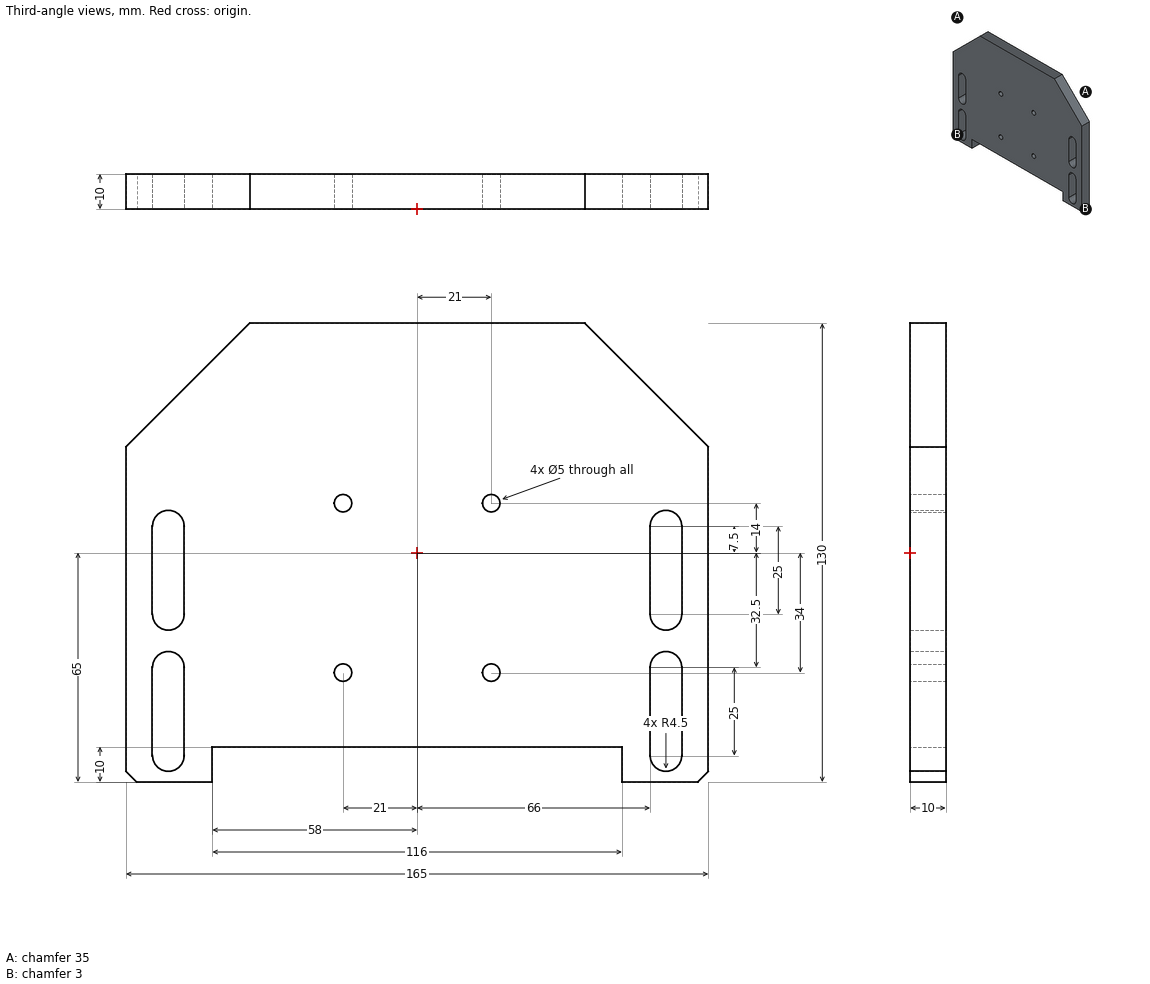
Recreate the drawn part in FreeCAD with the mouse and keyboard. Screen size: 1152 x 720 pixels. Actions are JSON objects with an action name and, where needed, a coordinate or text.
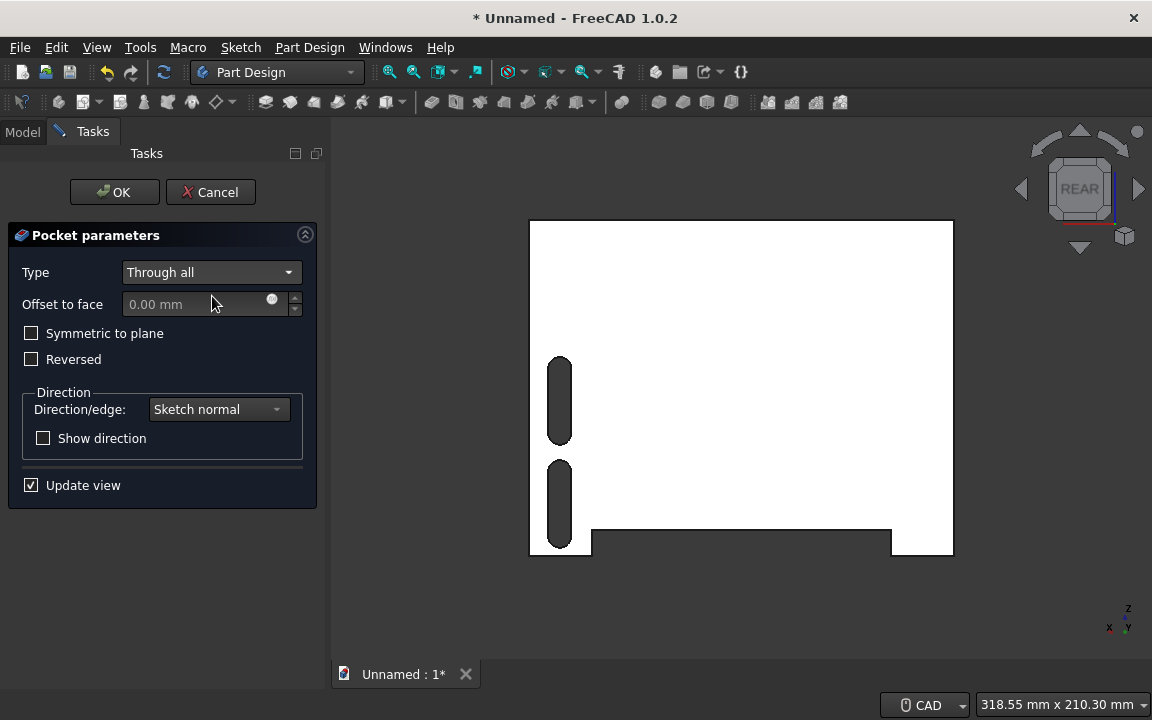
{"action": "left_click", "coordinate": [115, 192]}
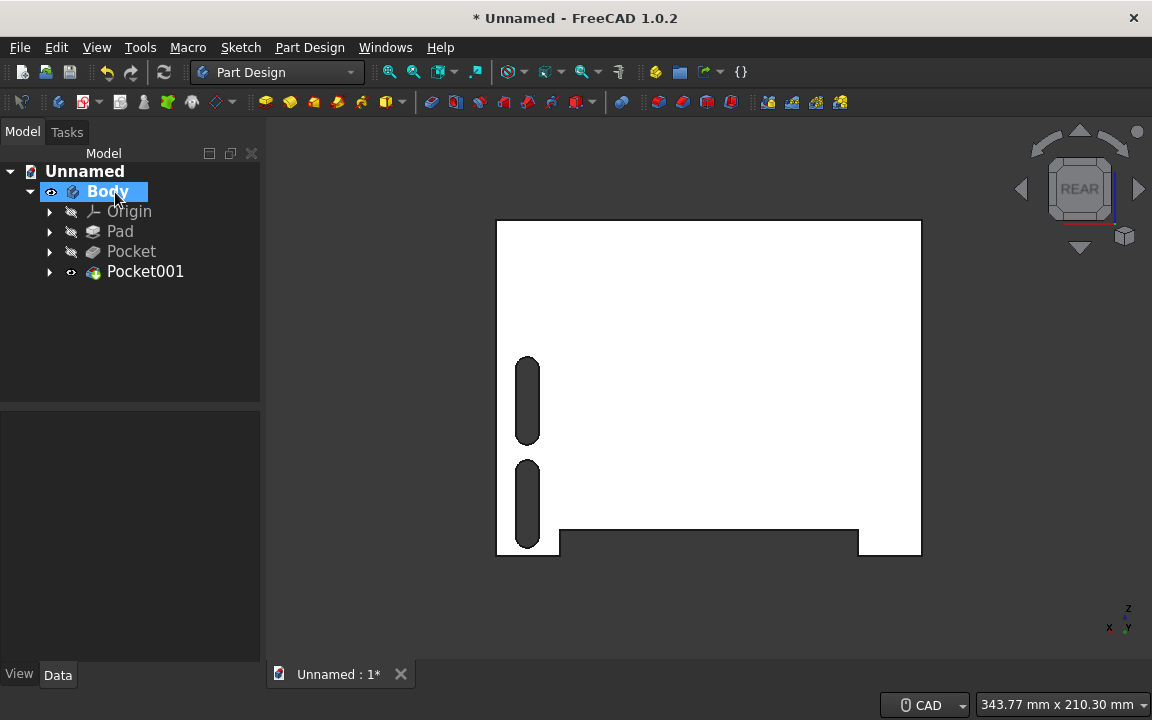
{"action": "key", "text": "0"}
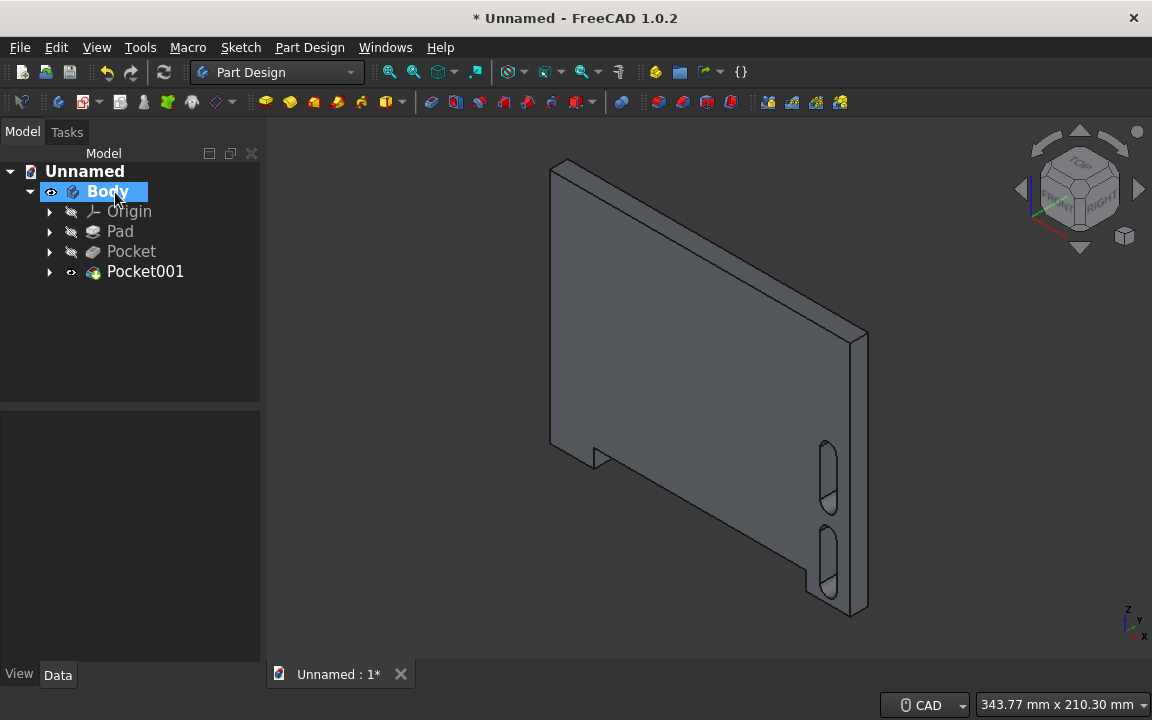
{"action": "left_click", "coordinate": [859, 337]}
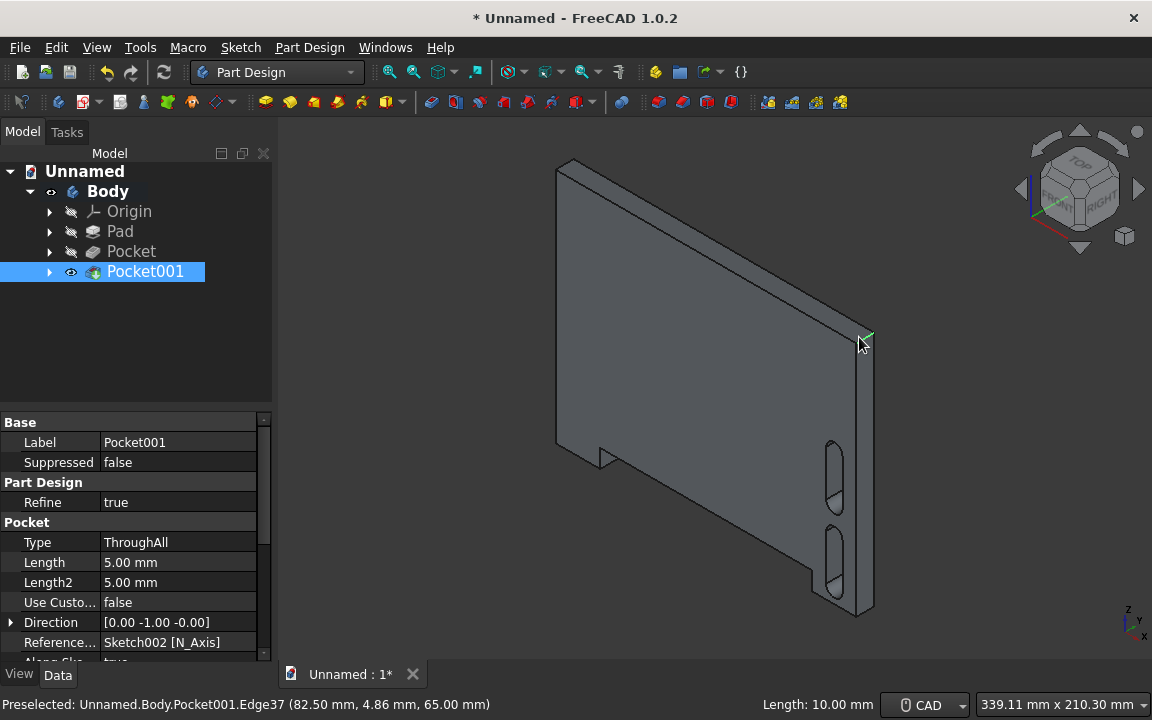
{"action": "key", "text": "2"}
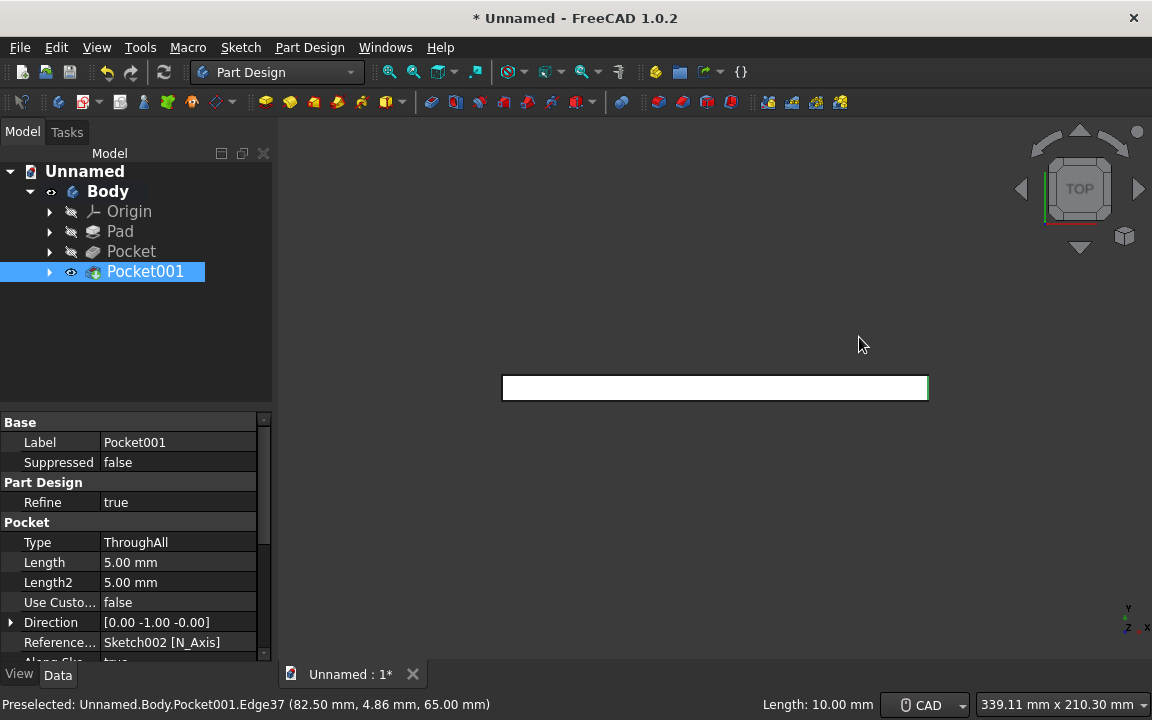
{"action": "left_click", "coordinate": [502, 387], "text": "ctrl"}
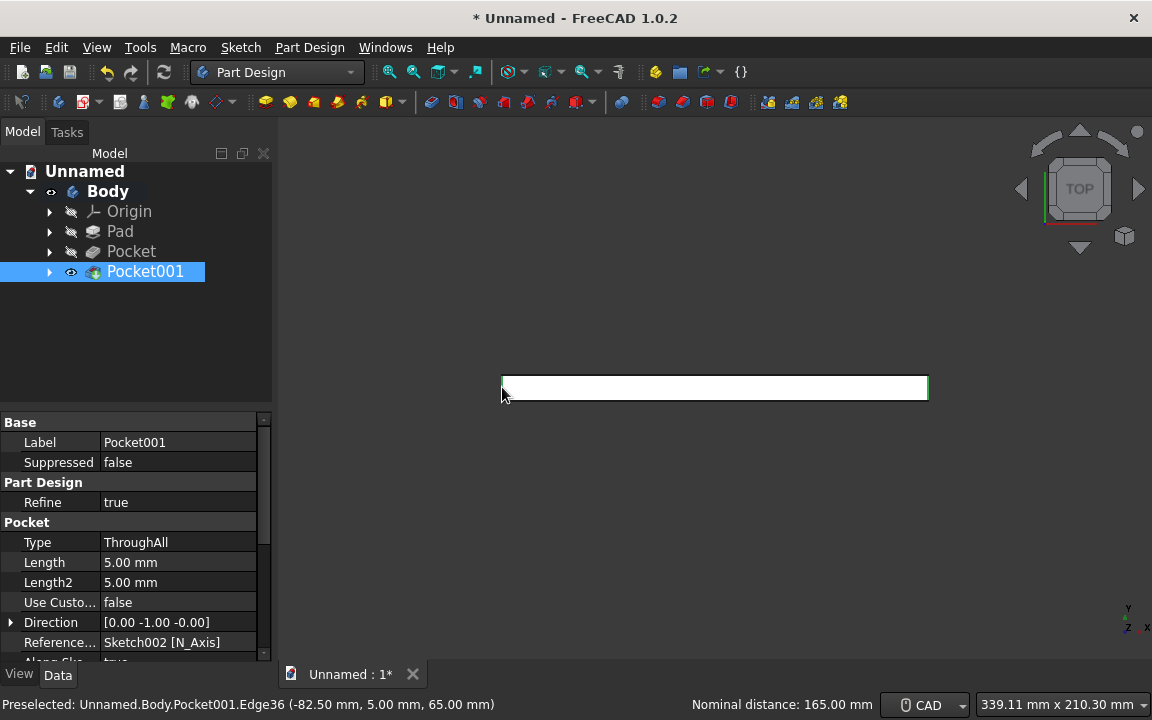
{"action": "left_click", "coordinate": [684, 102]}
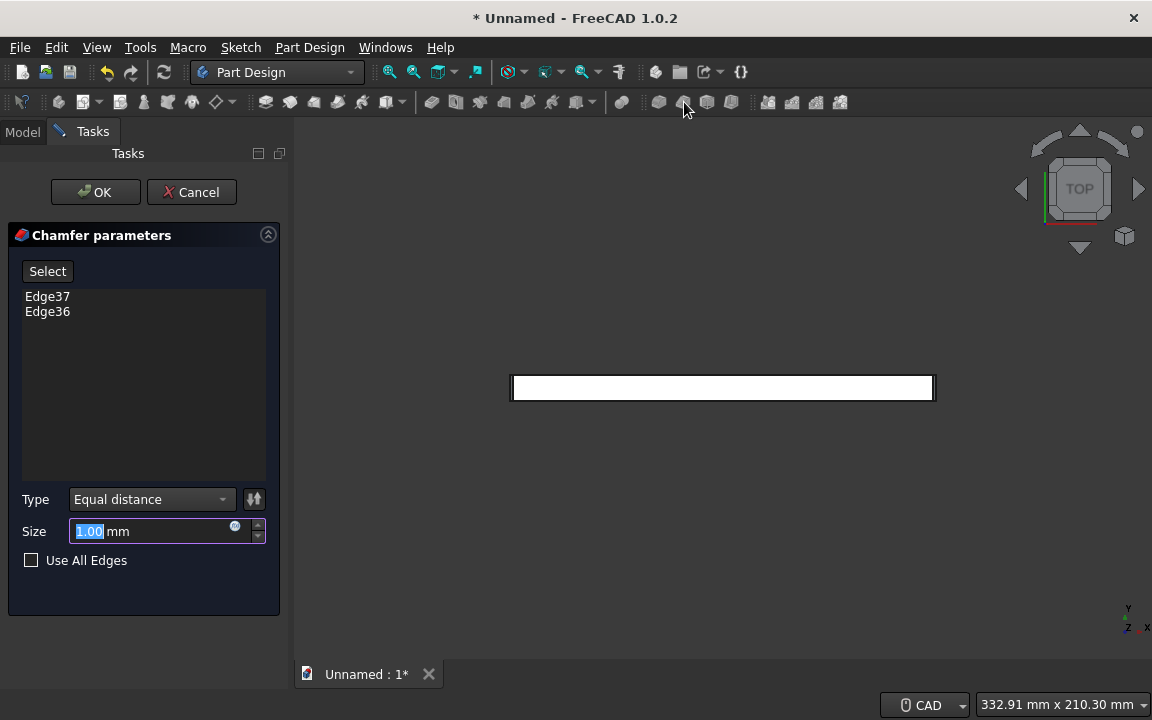
{"action": "type", "text": "35"}
{"action": "key", "text": "Tab"}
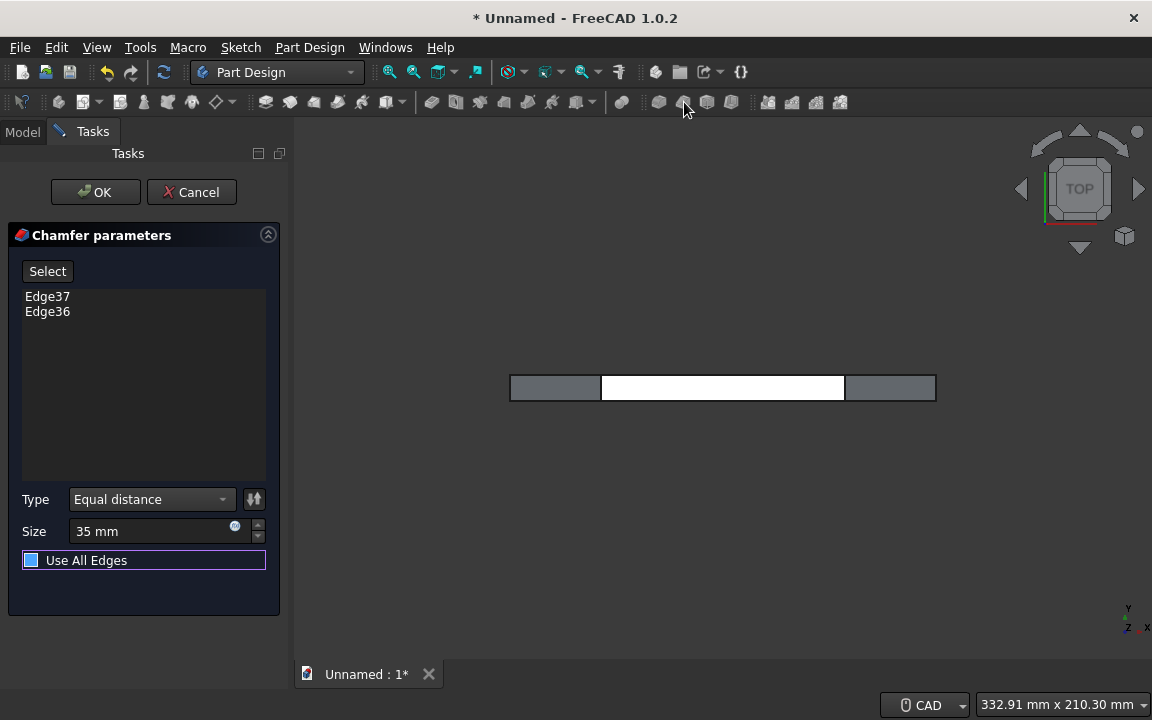
{"action": "left_click", "coordinate": [96, 192]}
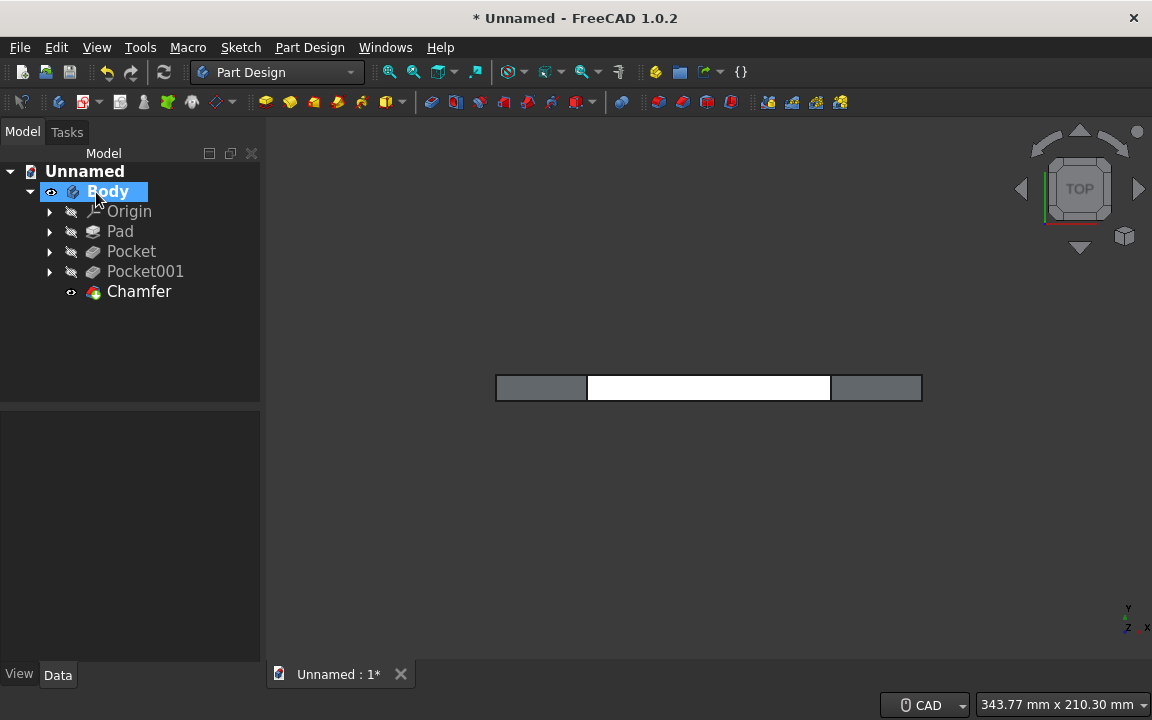
{"action": "key", "text": "4"}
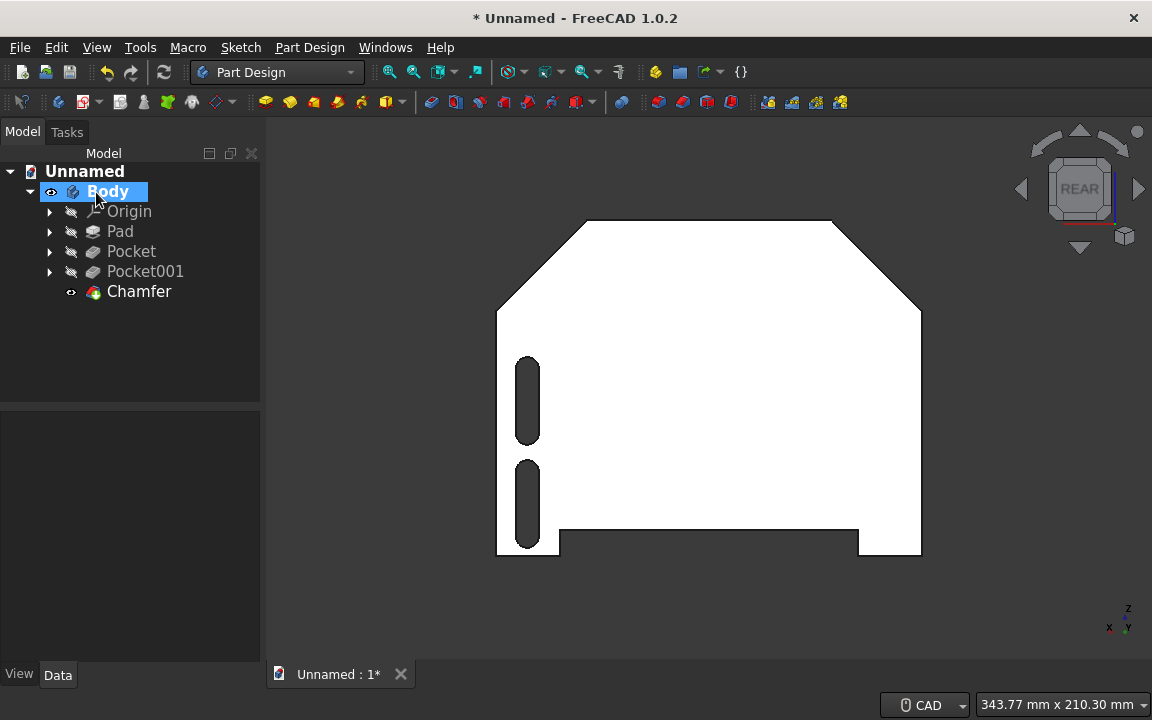
{"action": "left_click", "coordinate": [709, 387]}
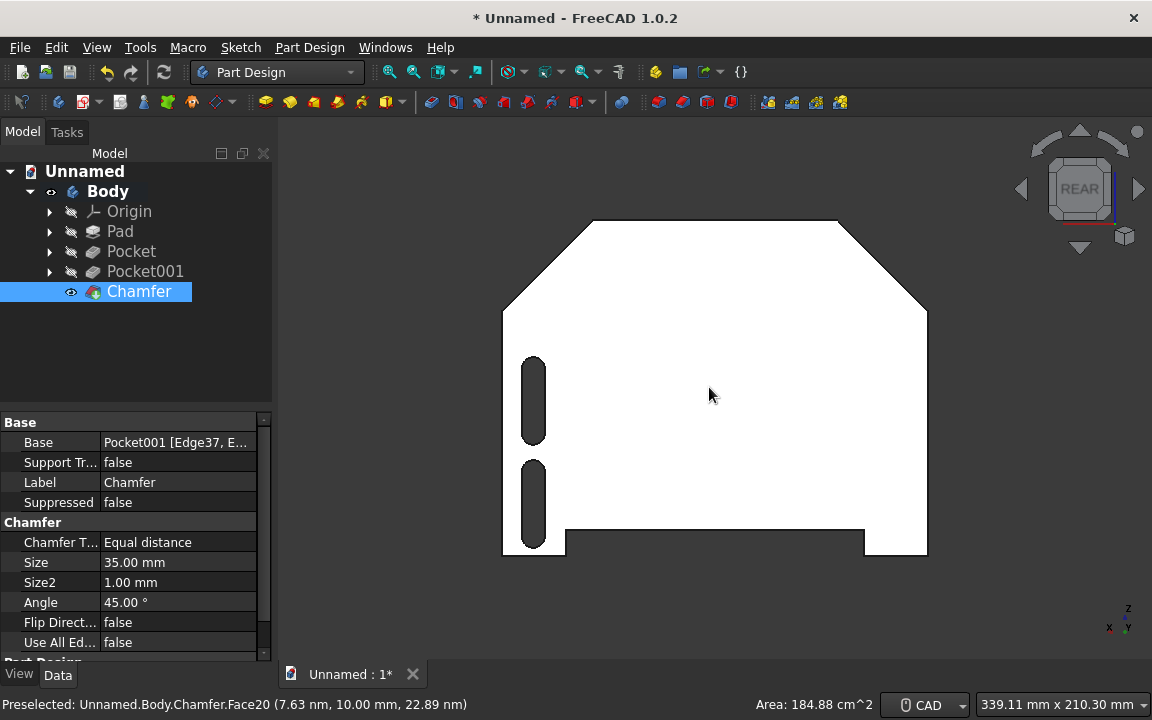
{"action": "left_click", "coordinate": [84, 102]}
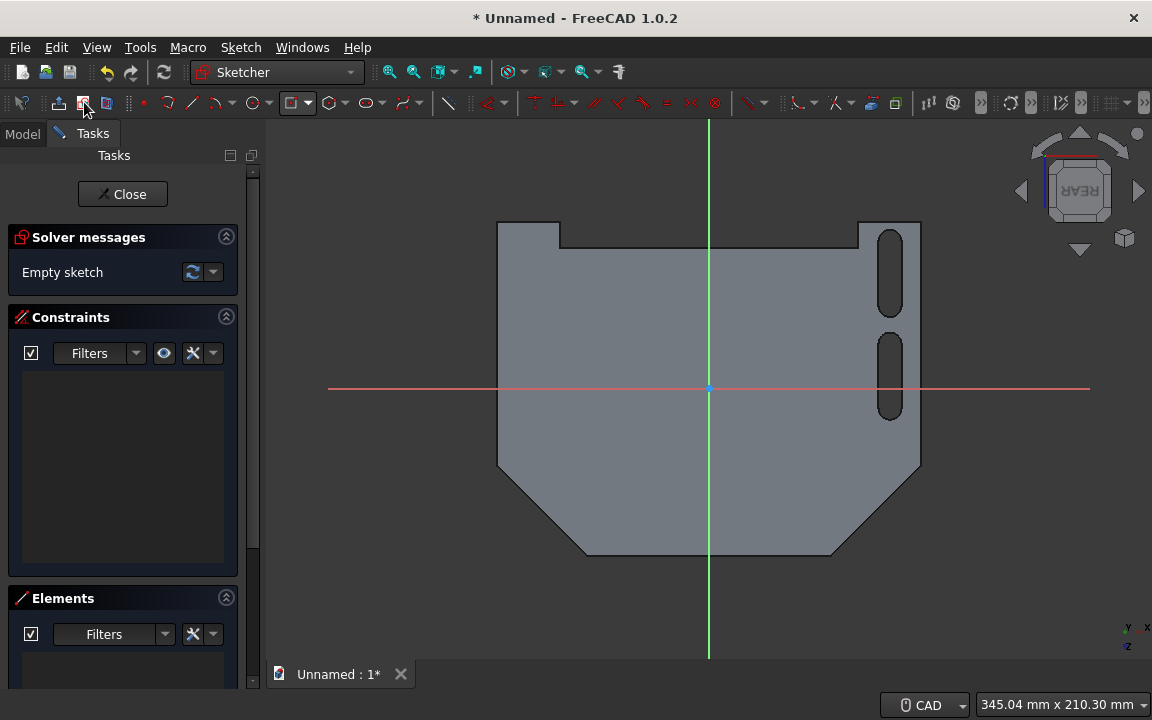
{"action": "scroll", "coordinate": [749, 348], "scroll_direction": "up", "scroll_amount": 5}